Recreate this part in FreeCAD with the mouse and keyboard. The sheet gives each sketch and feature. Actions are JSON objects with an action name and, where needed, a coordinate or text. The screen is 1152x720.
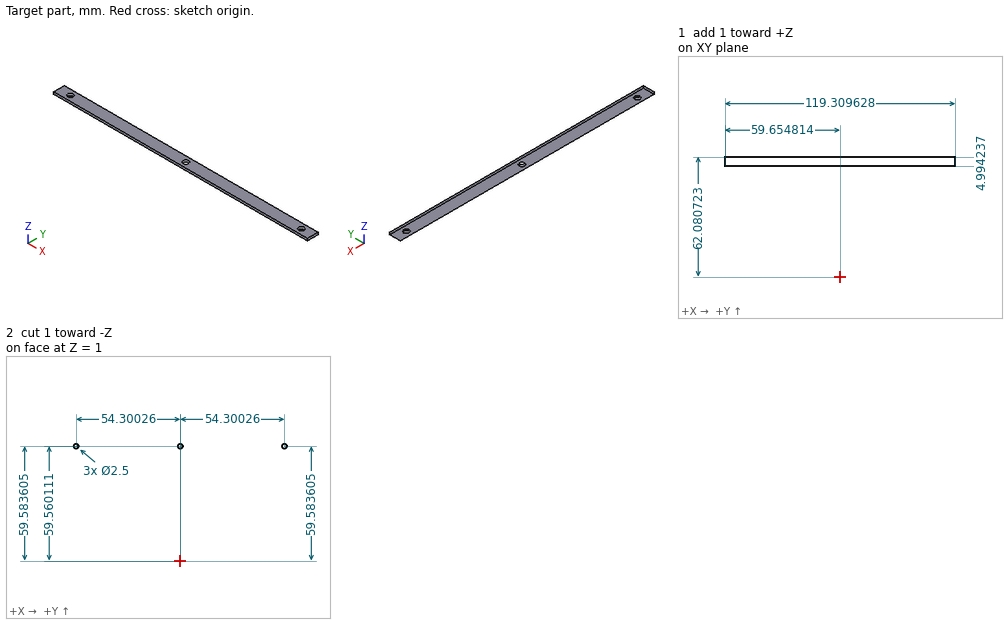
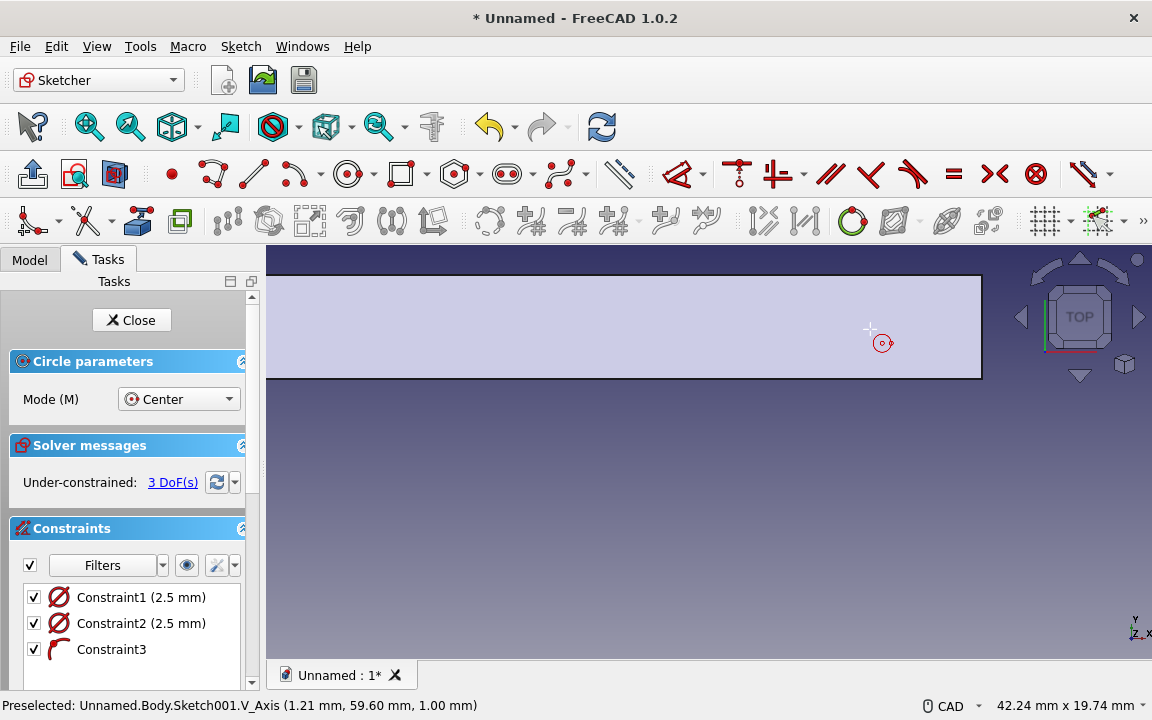
{"action": "scroll", "coordinate": [871, 329], "scroll_direction": "down", "scroll_amount": 8}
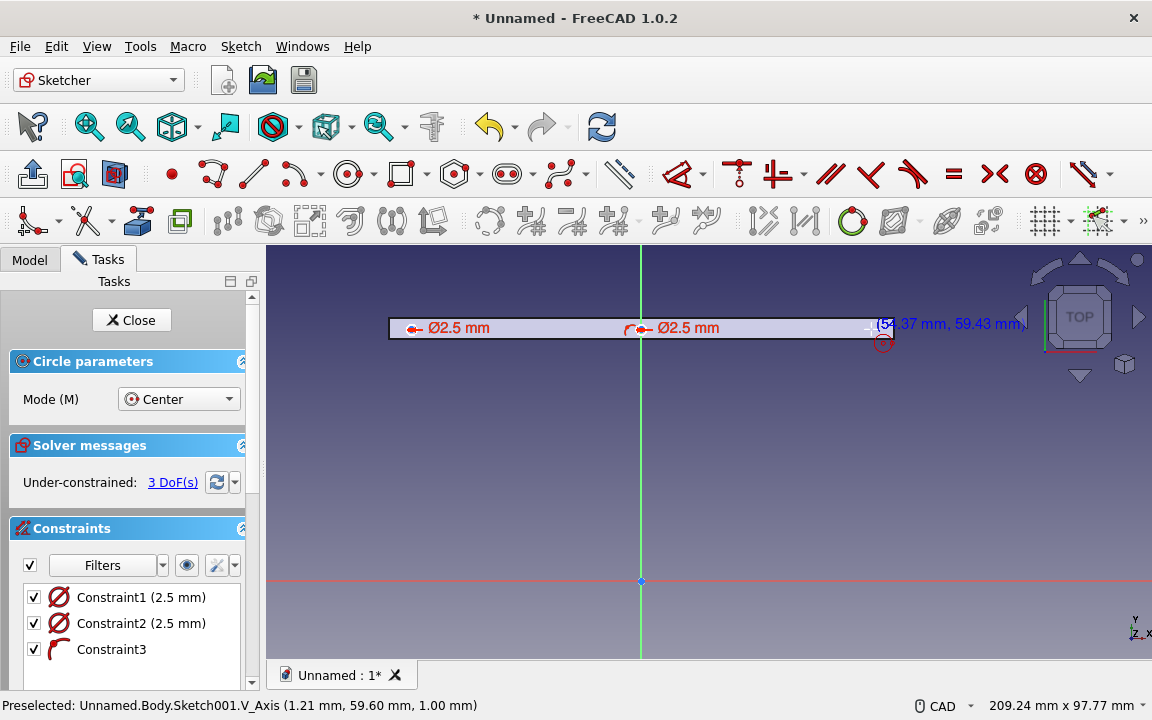
{"action": "left_click", "coordinate": [871, 329]}
{"action": "mouse_move", "coordinate": [875, 325]}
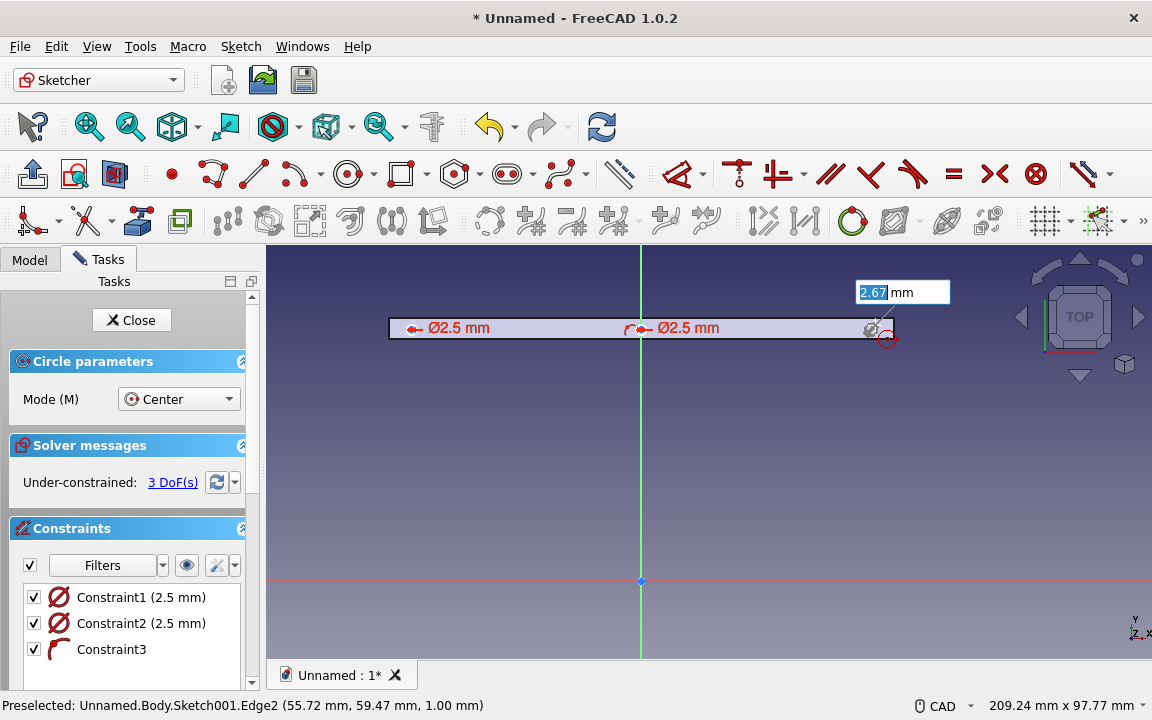
{"action": "type", "text": "2.5"}
{"action": "key", "text": "Return"}
{"action": "key", "text": "Escape"}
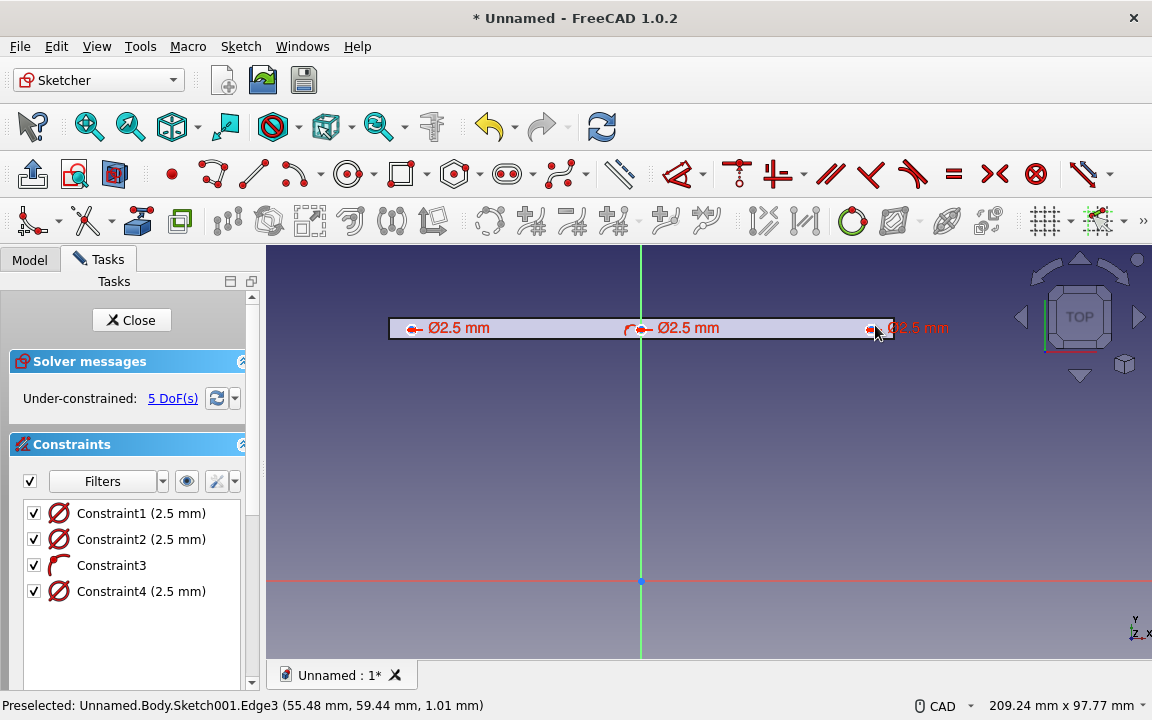
{"action": "key", "text": "d"}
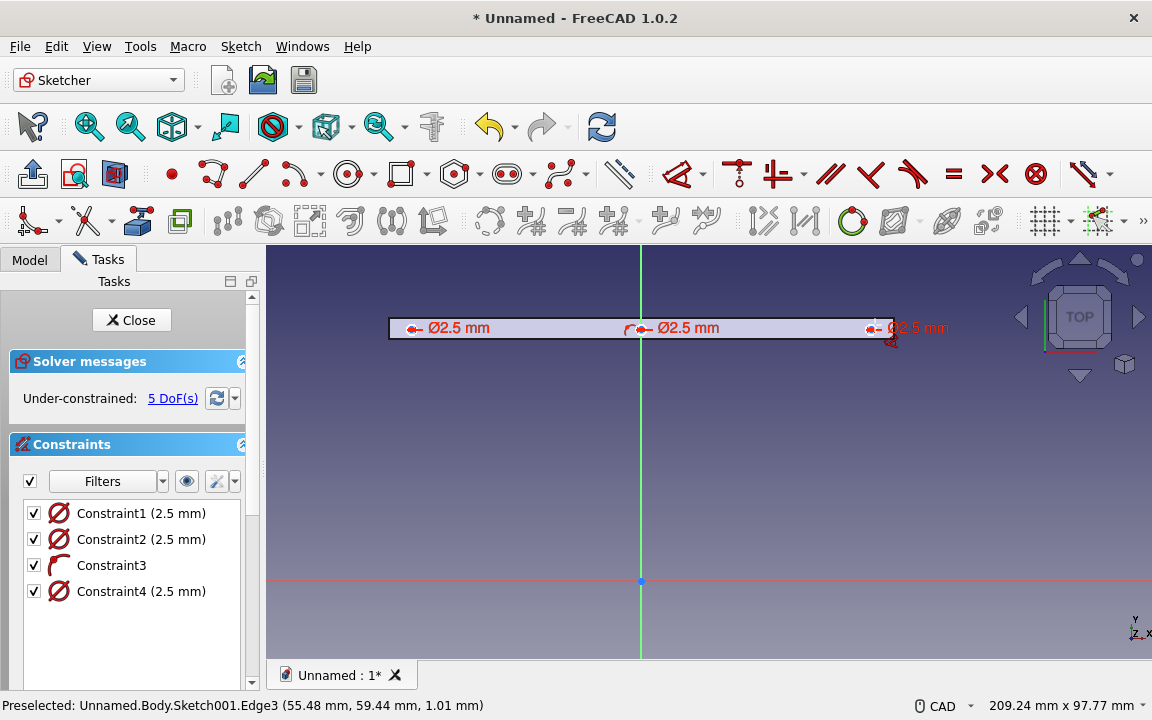
{"action": "left_click", "coordinate": [412, 330]}
{"action": "left_click", "coordinate": [527, 615]}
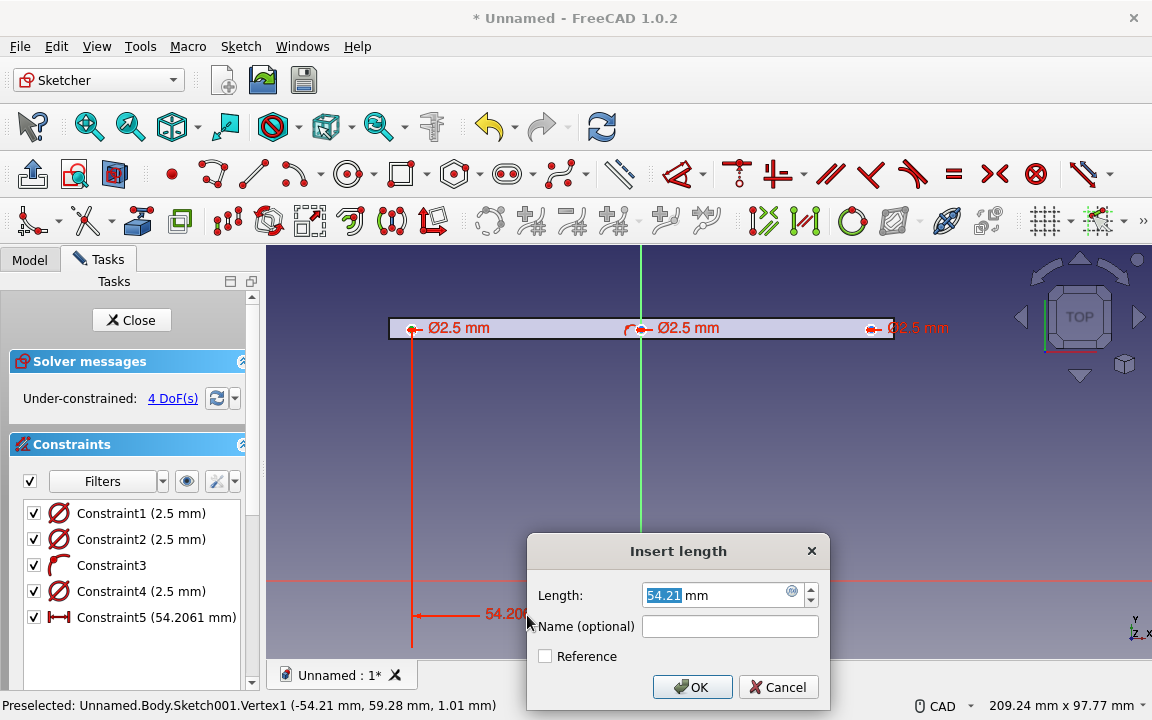
{"action": "type", "text": "54.30026"}
{"action": "key", "text": "Return"}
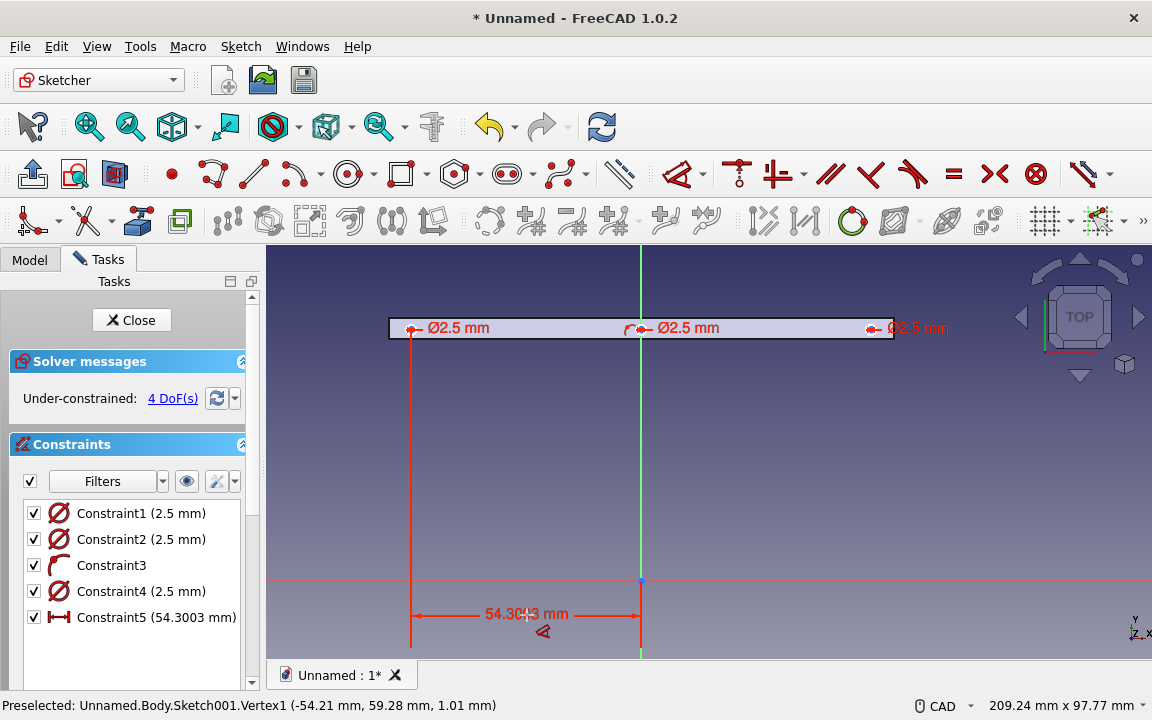
{"action": "left_click", "coordinate": [871, 330]}
{"action": "left_click", "coordinate": [756, 615]}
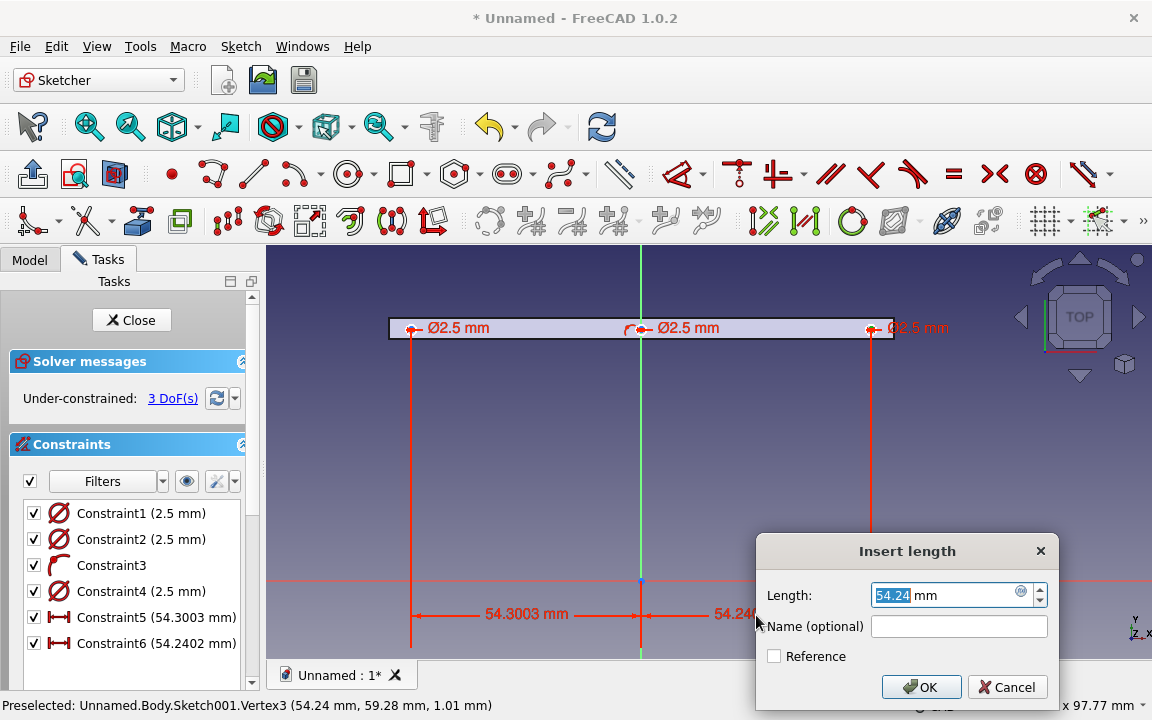
{"action": "type", "text": "54.30026"}
{"action": "key", "text": "Return"}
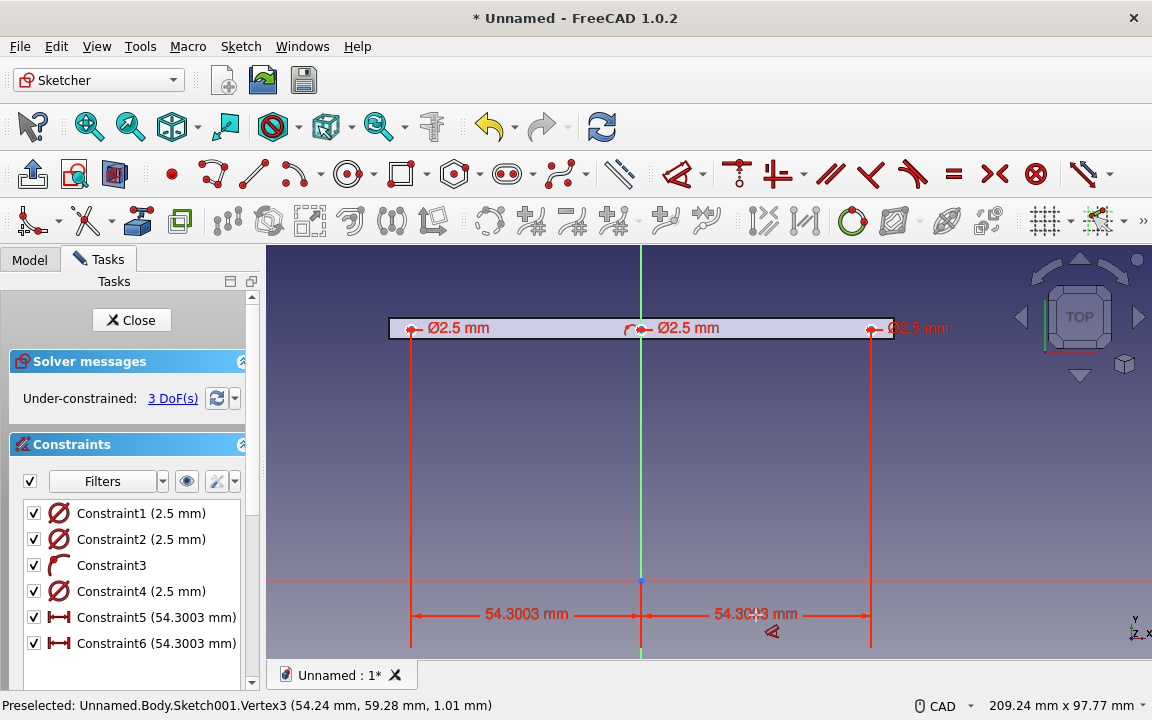
{"action": "left_click", "coordinate": [411, 330]}
{"action": "left_click", "coordinate": [377, 456]}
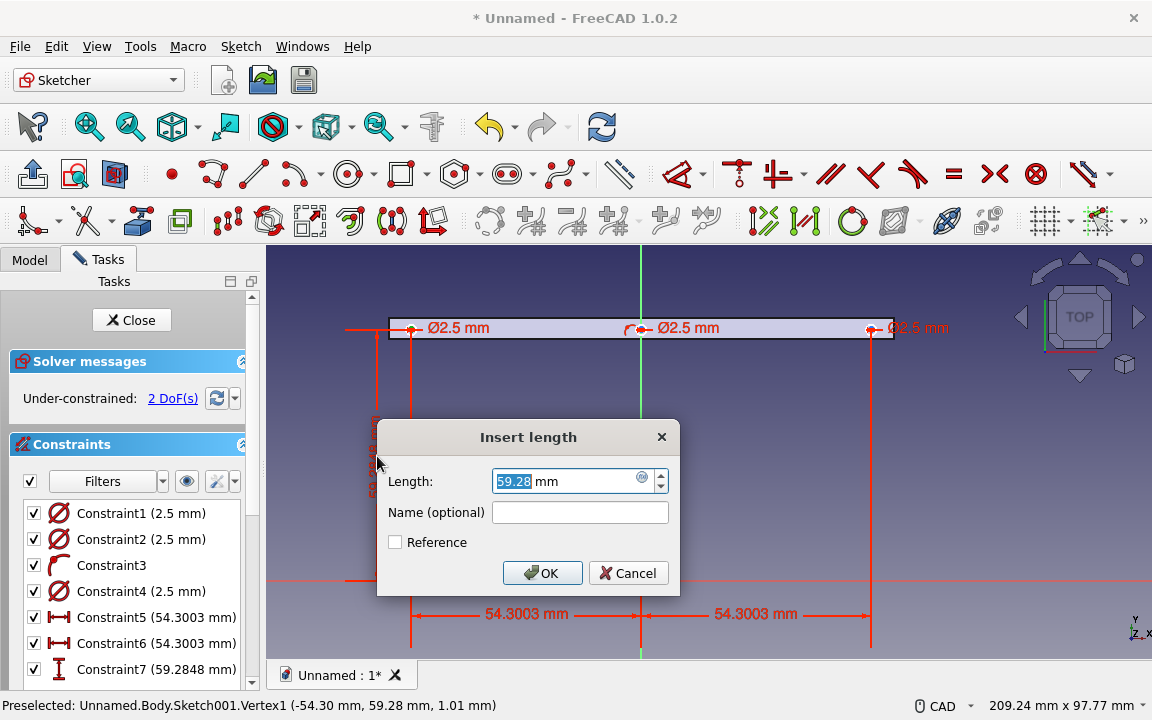
{"action": "type", "text": "59.583605"}
{"action": "key", "text": "Return"}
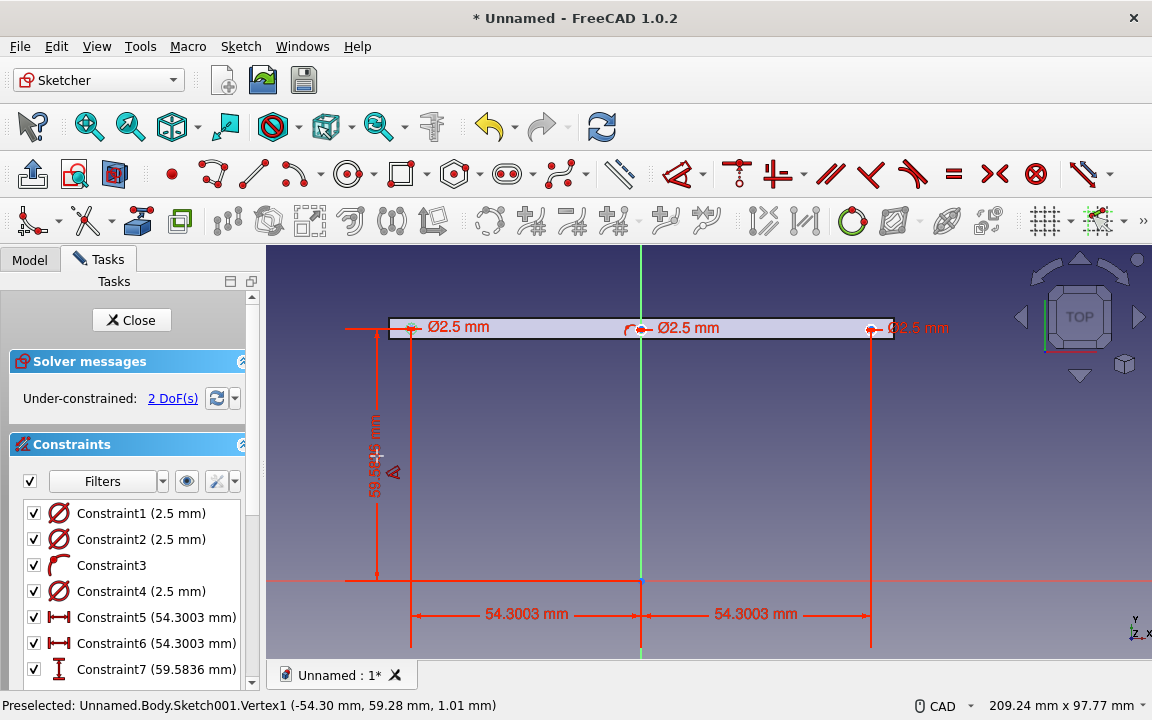
{"action": "left_click", "coordinate": [641, 330]}
{"action": "left_click", "coordinate": [675, 456]}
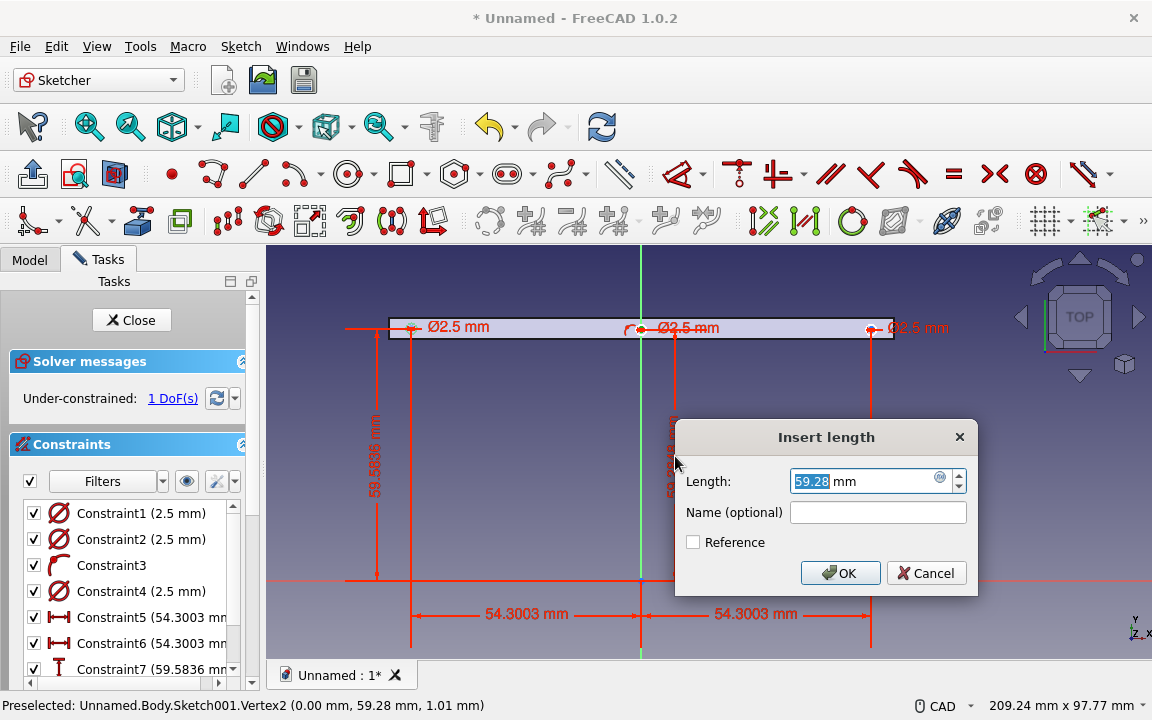
{"action": "type", "text": "59.560111"}
{"action": "key", "text": "Return"}